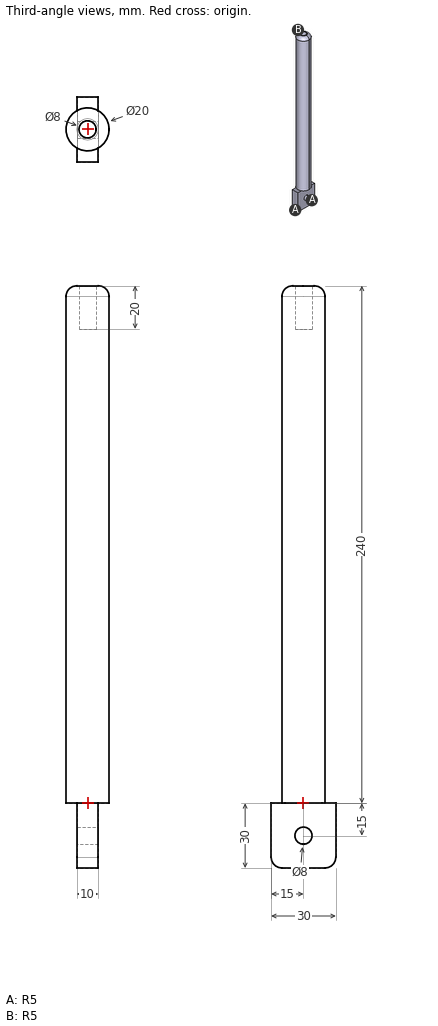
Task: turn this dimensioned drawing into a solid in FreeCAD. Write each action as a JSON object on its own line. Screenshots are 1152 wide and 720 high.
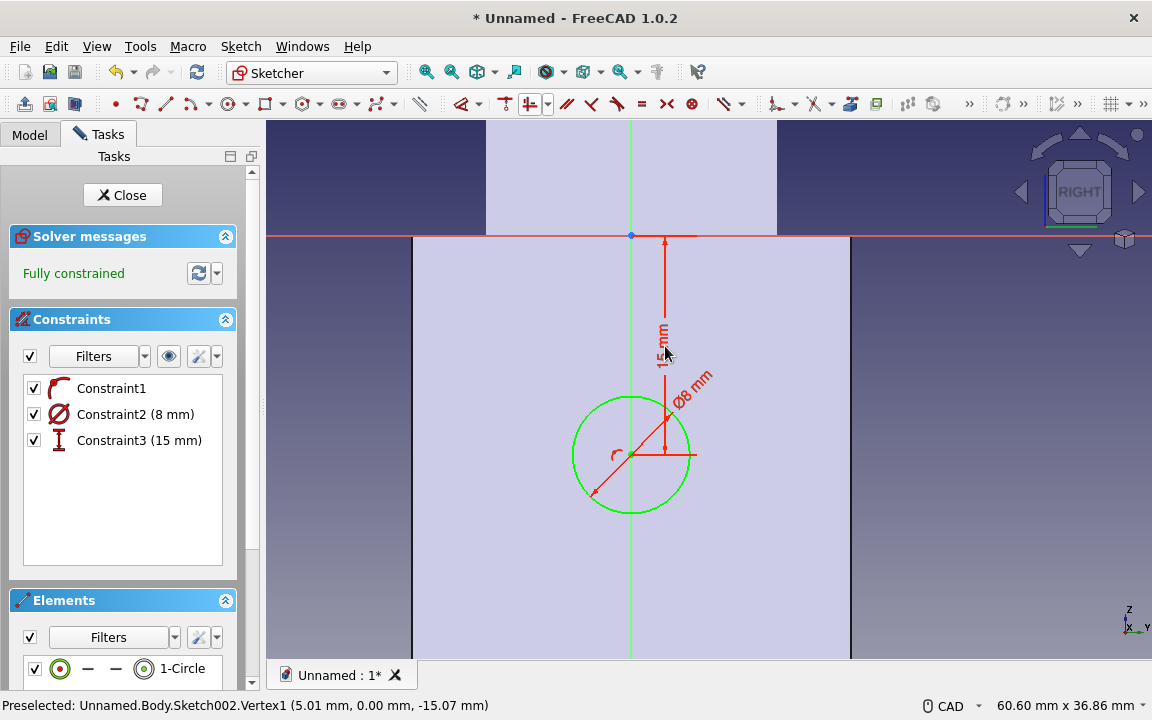
{"action": "left_click", "coordinate": [123, 195]}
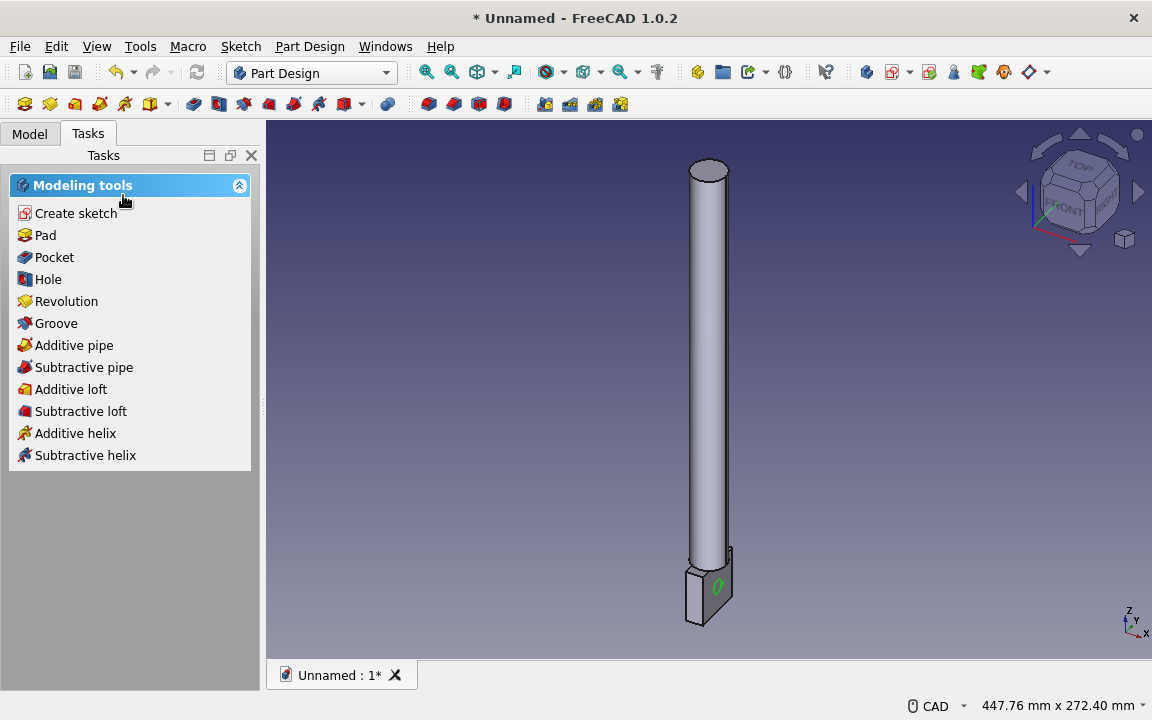
{"action": "left_click", "coordinate": [194, 104]}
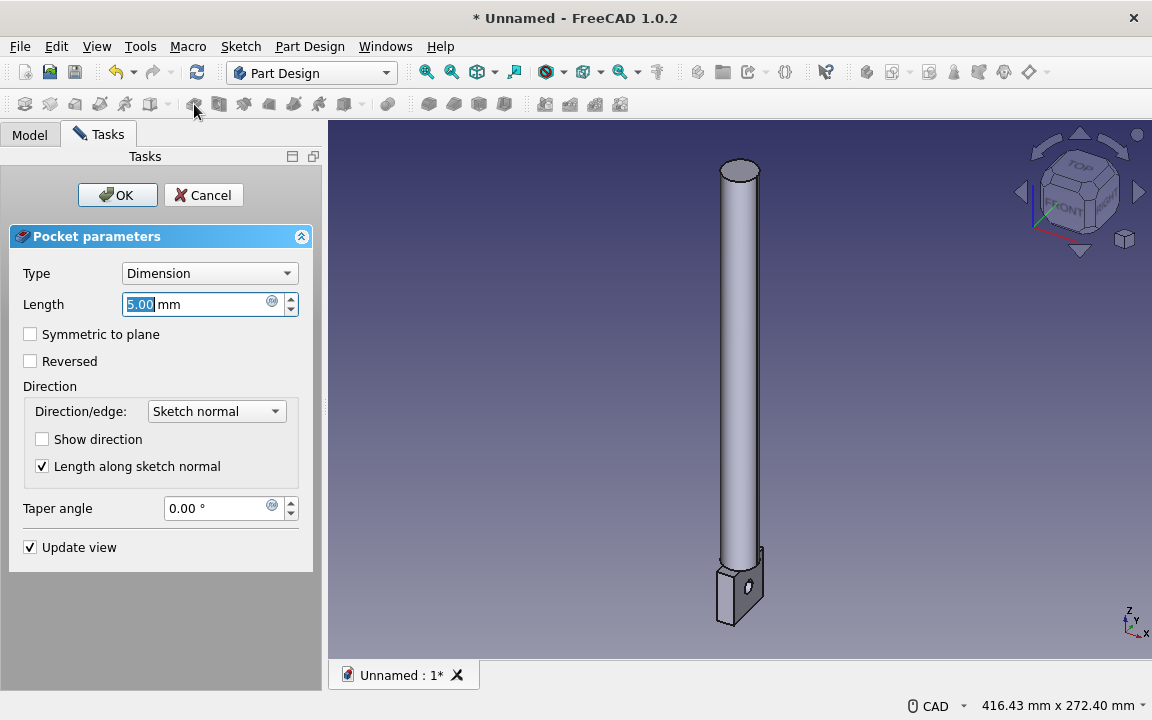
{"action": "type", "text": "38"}
{"action": "key", "text": "Tab"}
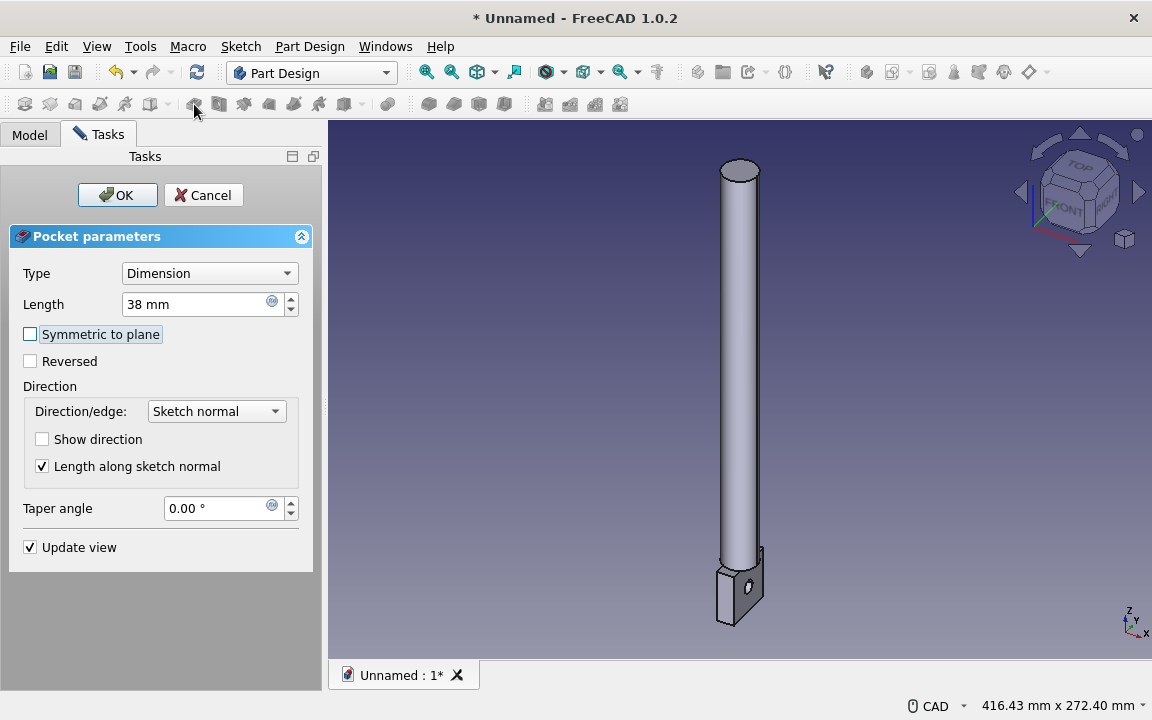
{"action": "left_click", "coordinate": [118, 195]}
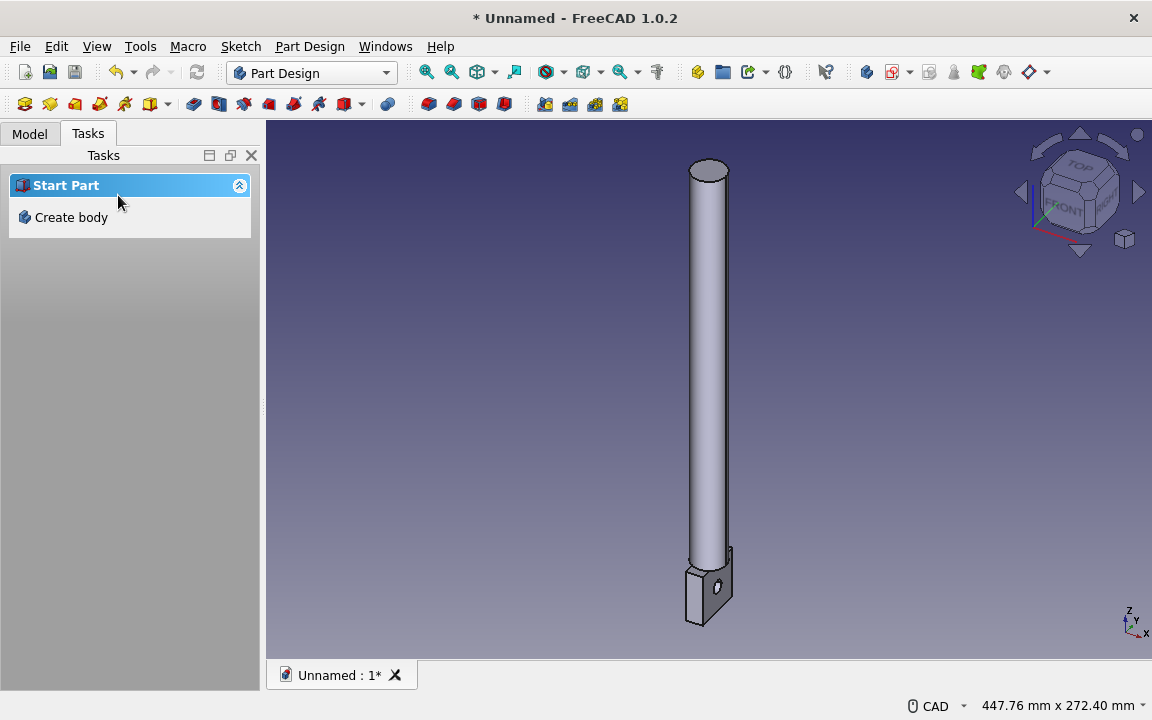
{"action": "scroll", "coordinate": [694, 622], "scroll_direction": "up", "scroll_amount": 4}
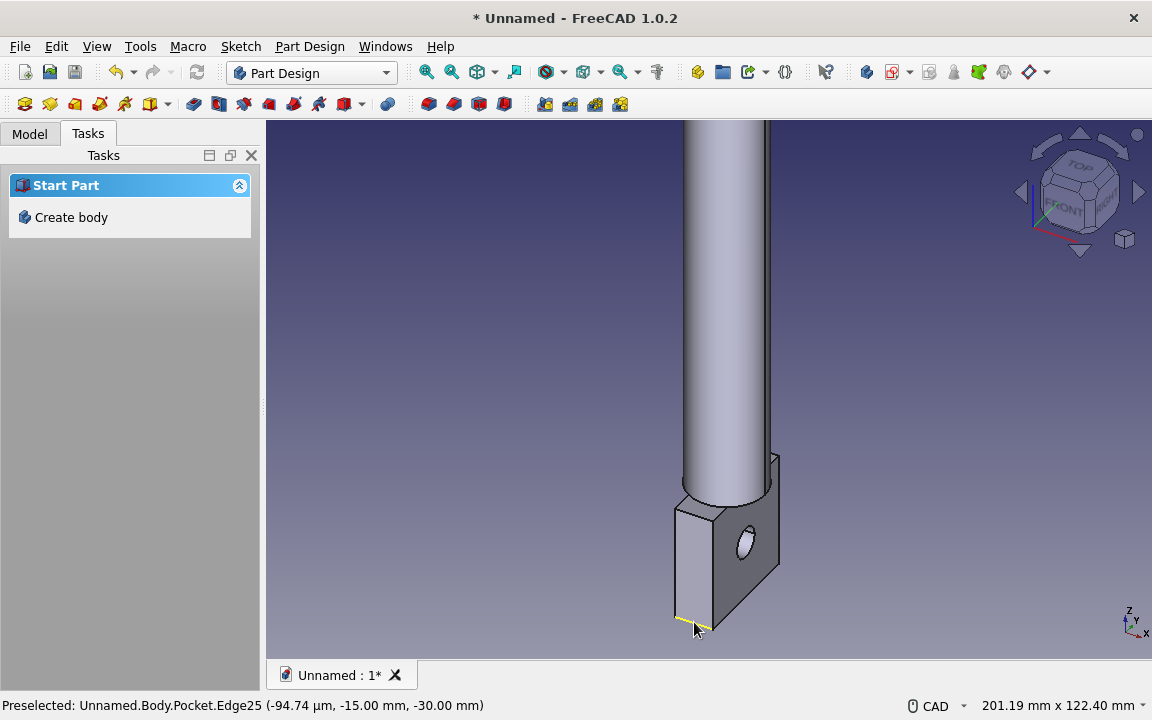
{"action": "left_click", "coordinate": [427, 72]}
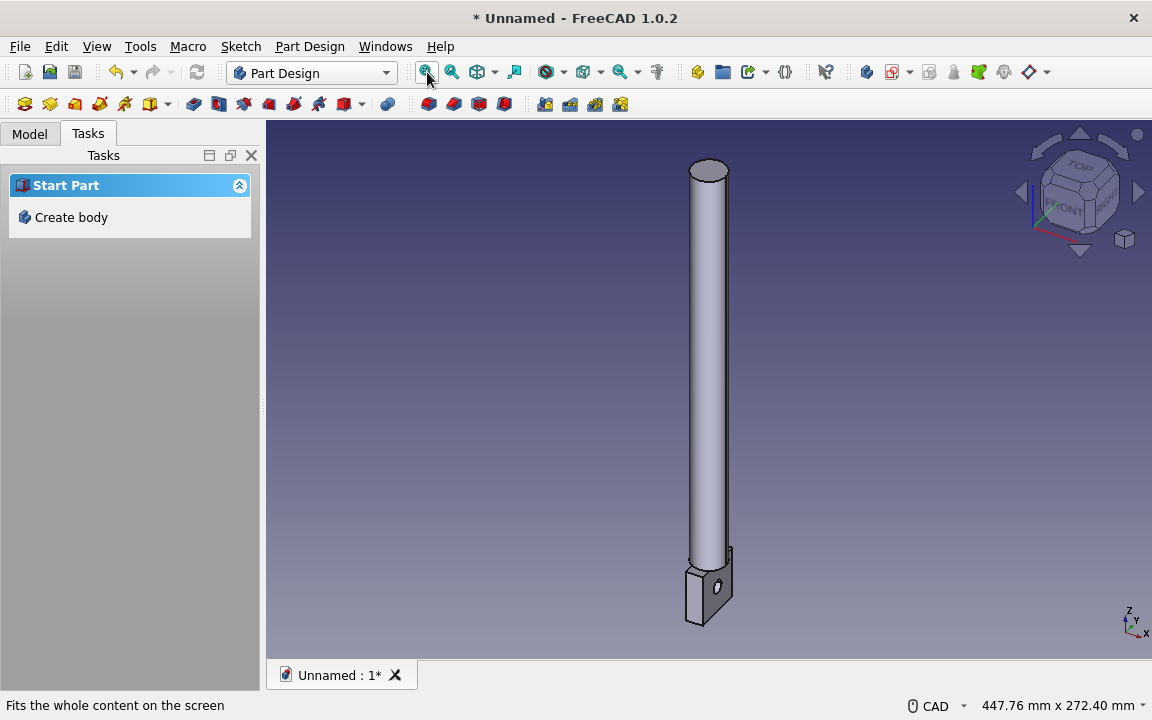
{"action": "key", "text": "0"}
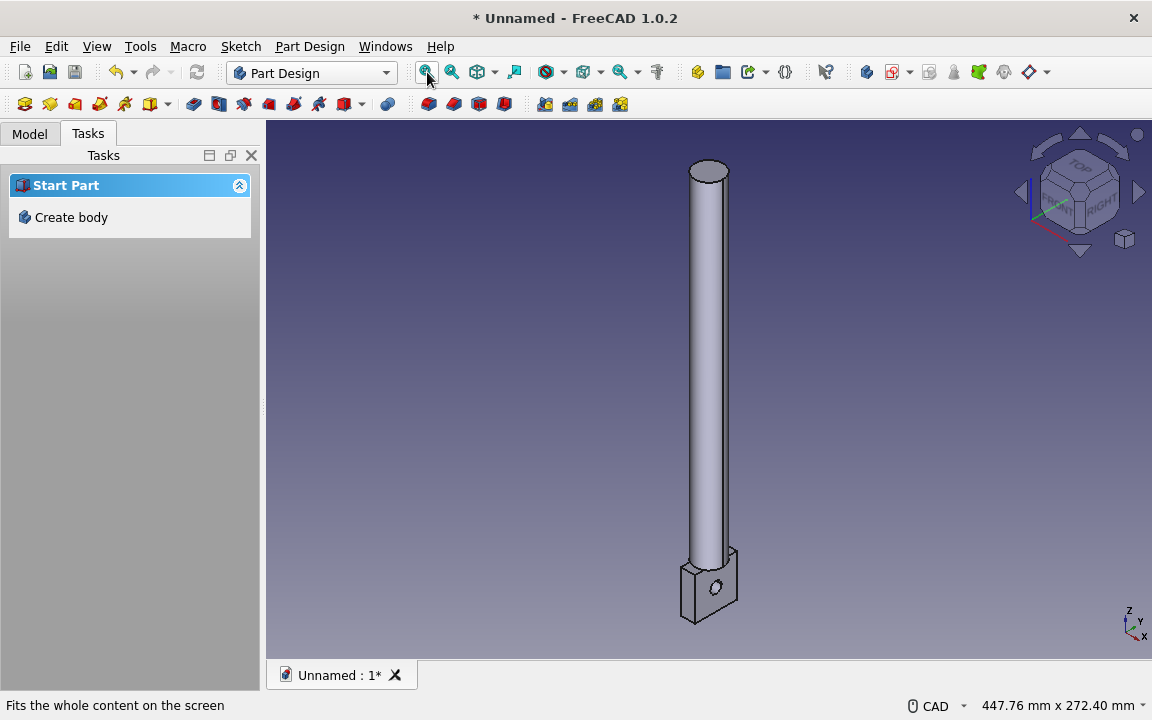
{"action": "scroll", "coordinate": [688, 619], "scroll_direction": "up", "scroll_amount": 4}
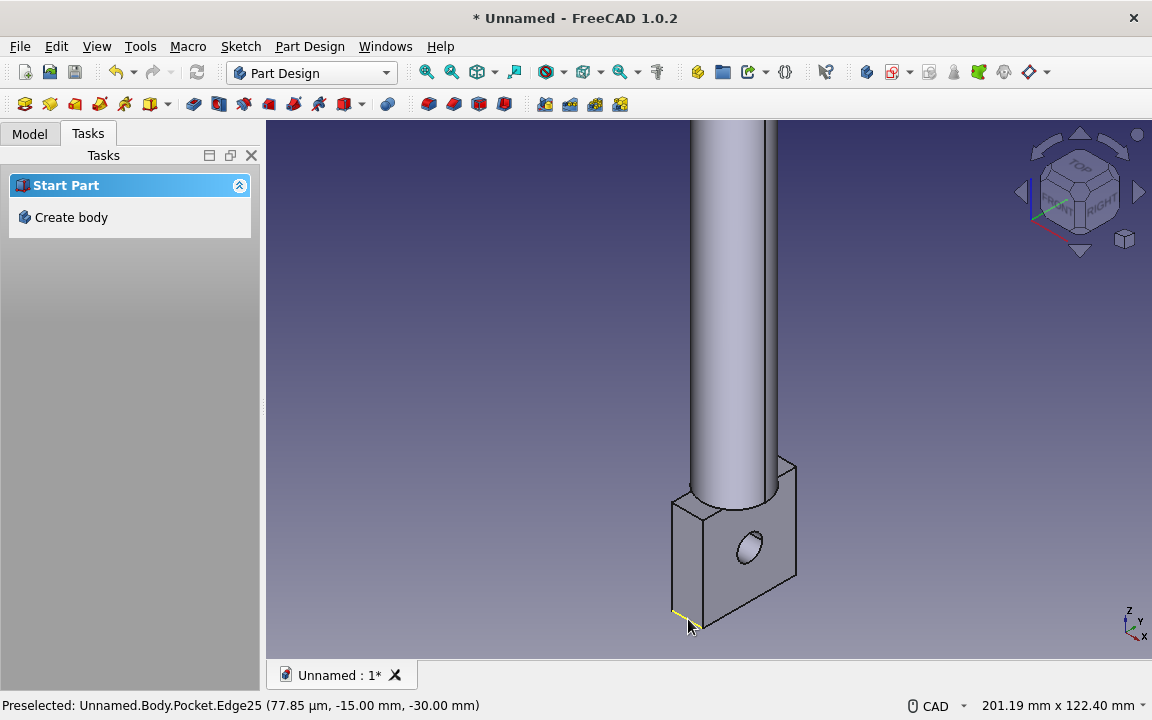
{"action": "left_click", "coordinate": [427, 72]}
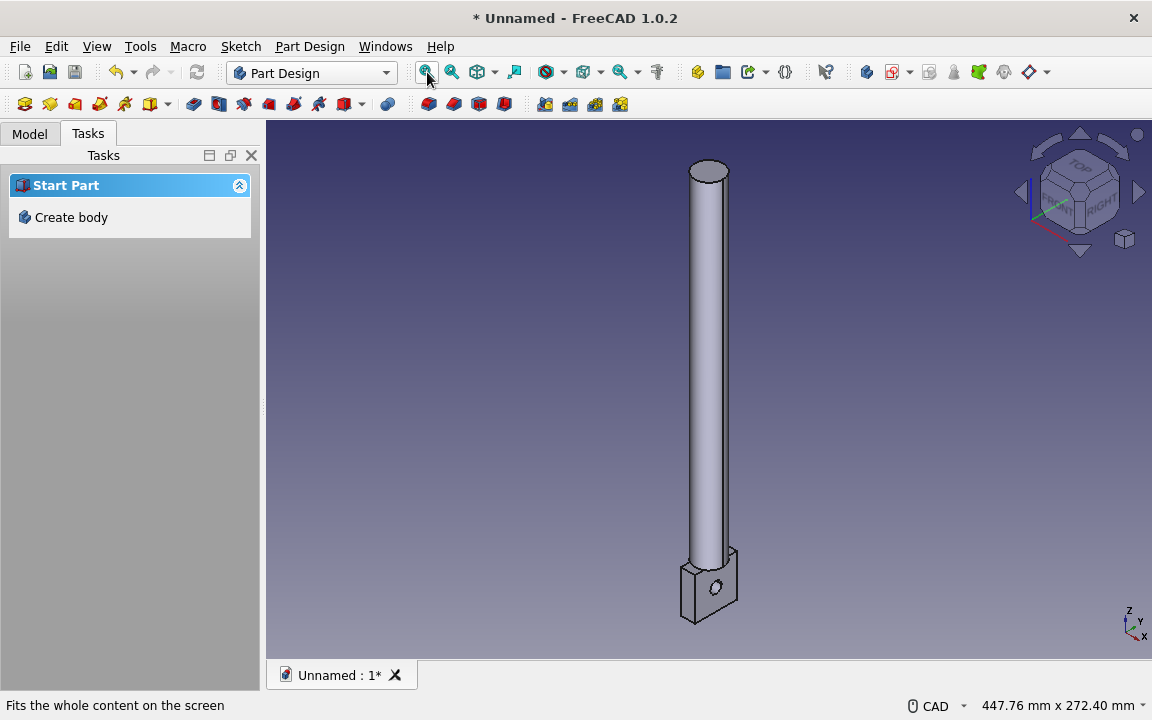
{"action": "key", "text": "2"}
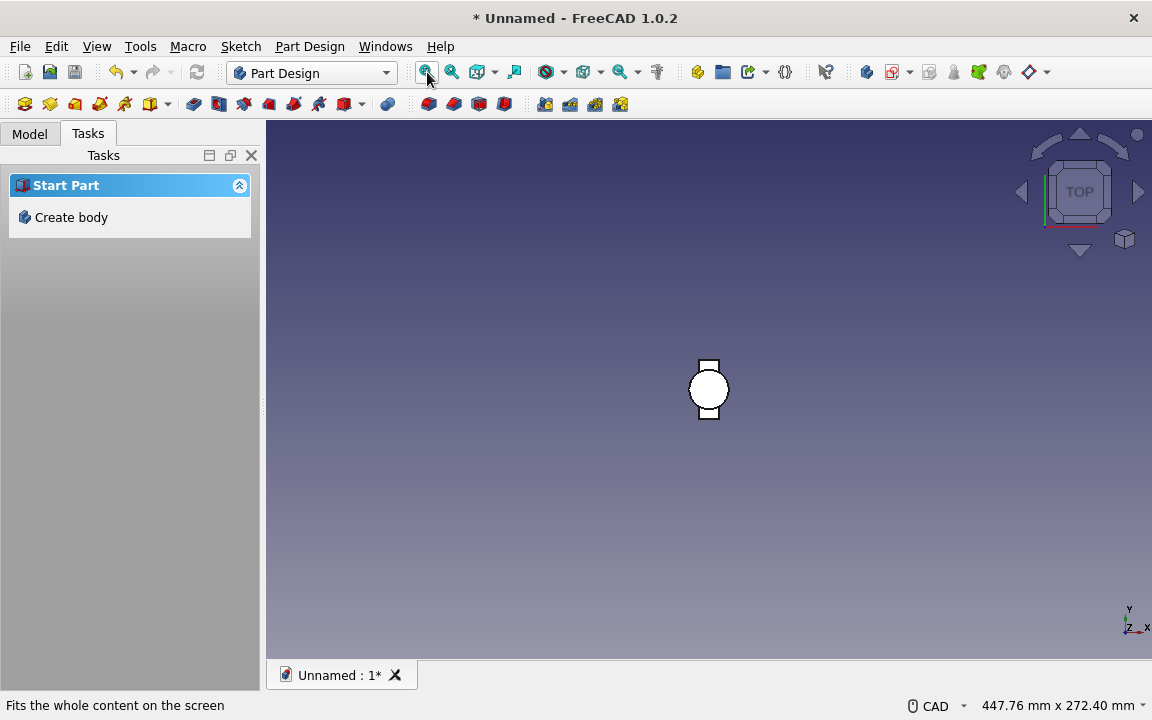
{"action": "left_click", "coordinate": [427, 72]}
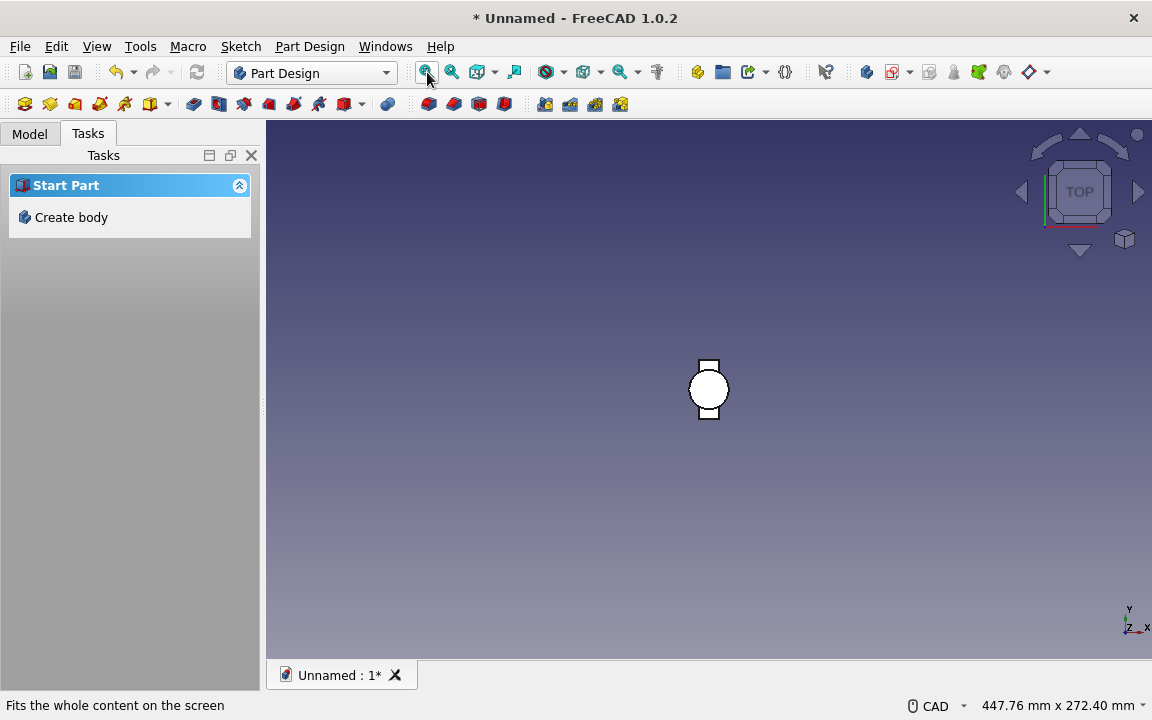
{"action": "scroll", "coordinate": [709, 418], "scroll_direction": "up", "scroll_amount": 4}